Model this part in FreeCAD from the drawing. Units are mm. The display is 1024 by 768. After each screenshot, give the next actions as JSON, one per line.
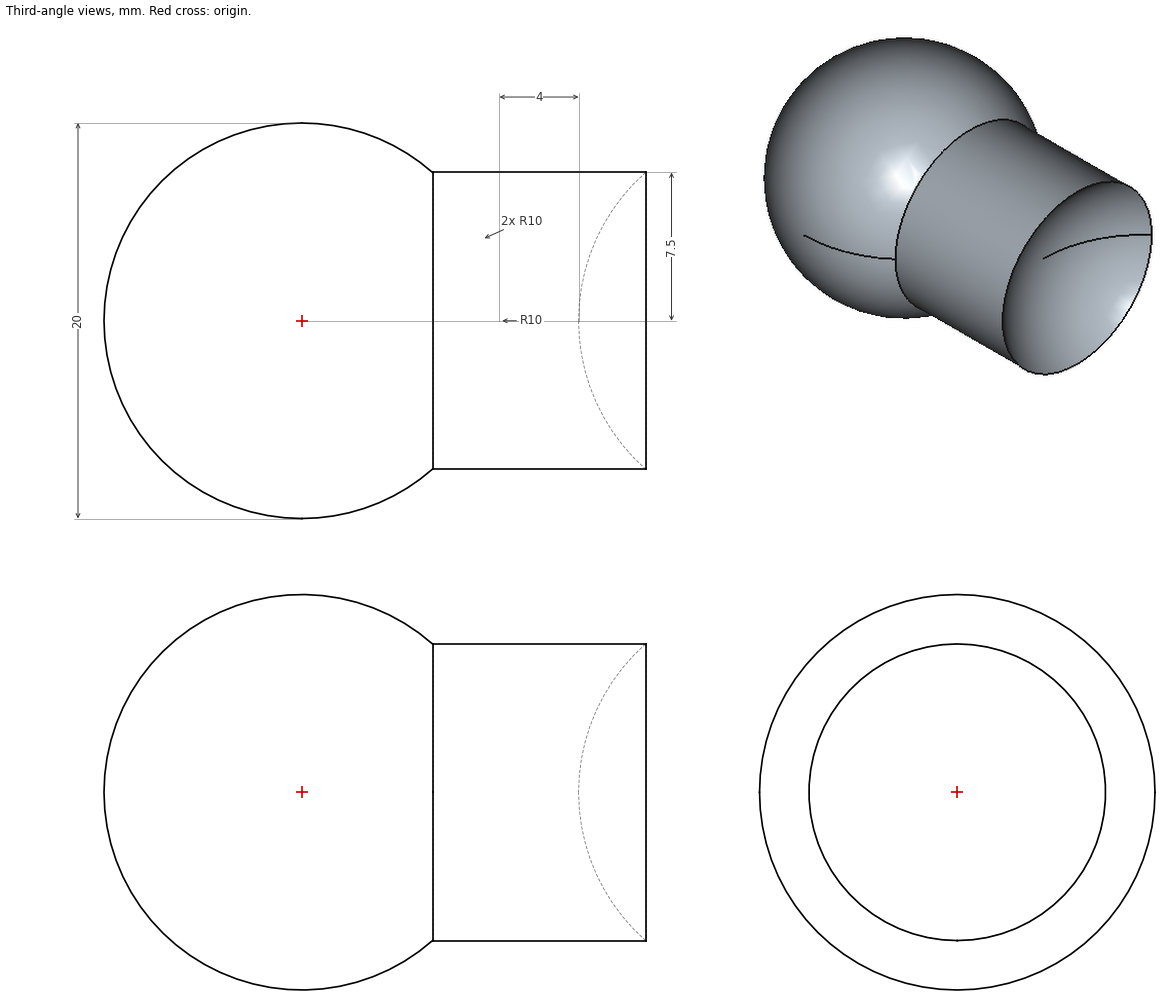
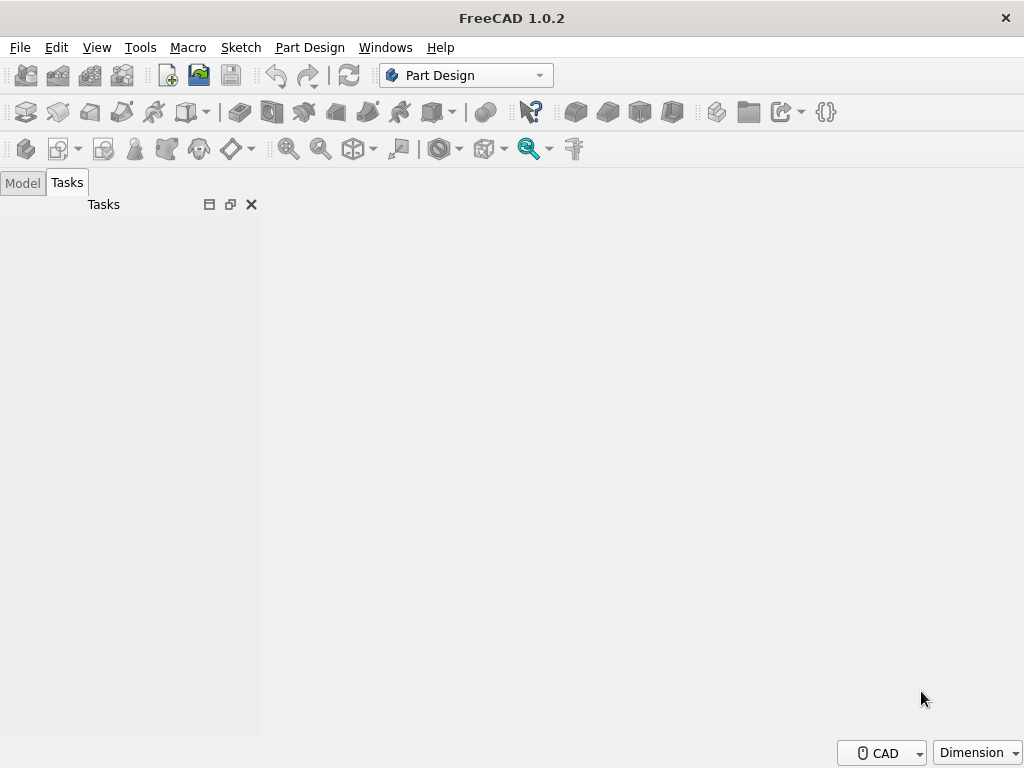
{"action": "key", "text": "ctrl+n"}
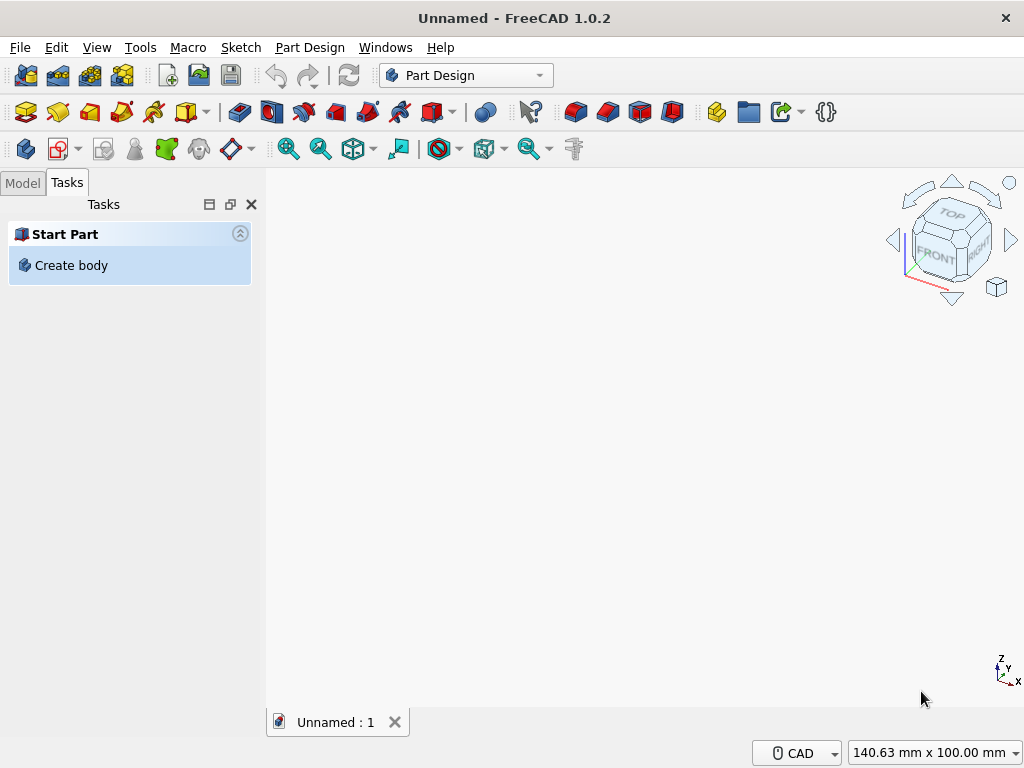
{"action": "left_click", "coordinate": [58, 150]}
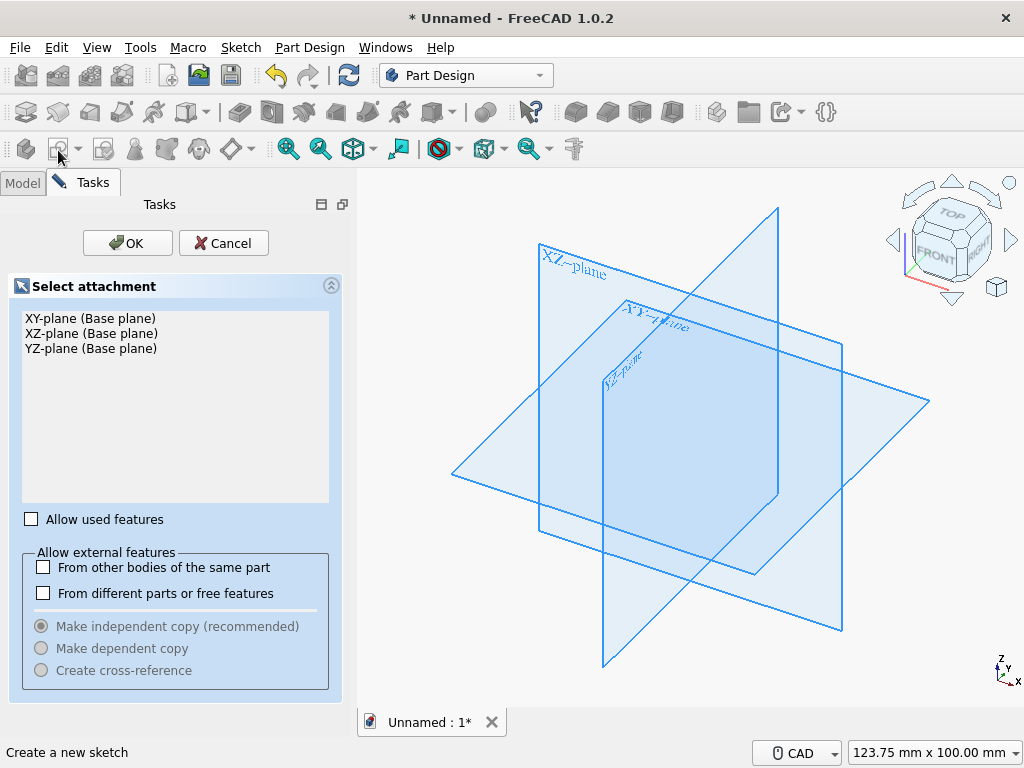
{"action": "left_click", "coordinate": [82, 318]}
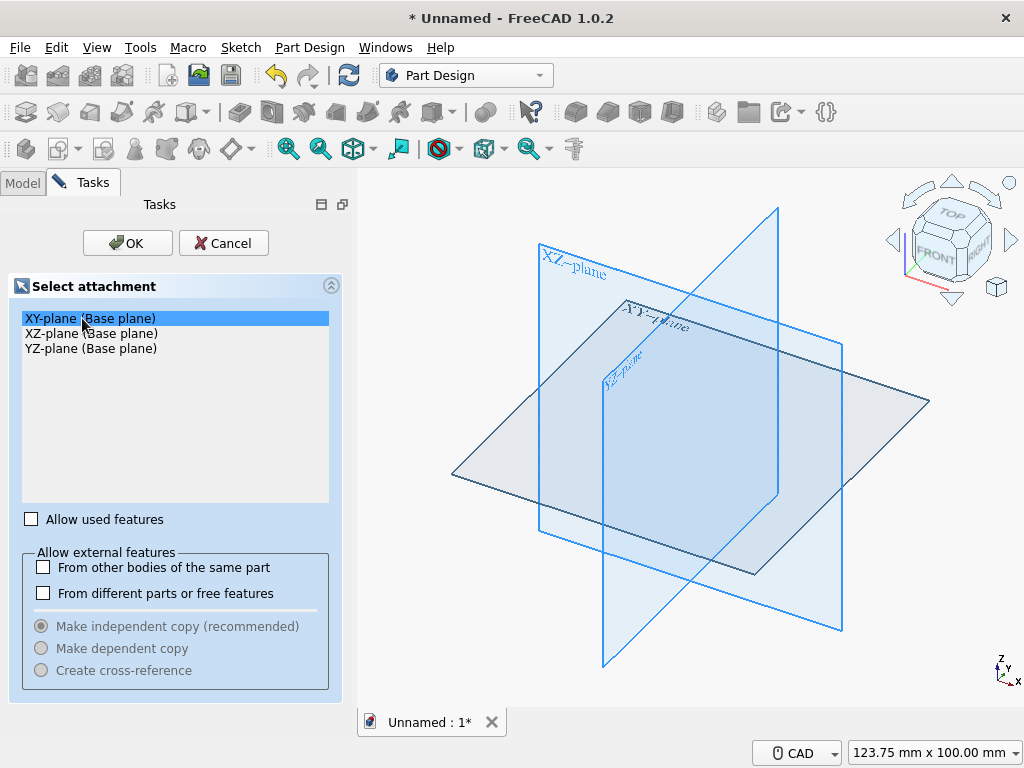
{"action": "left_click", "coordinate": [128, 243]}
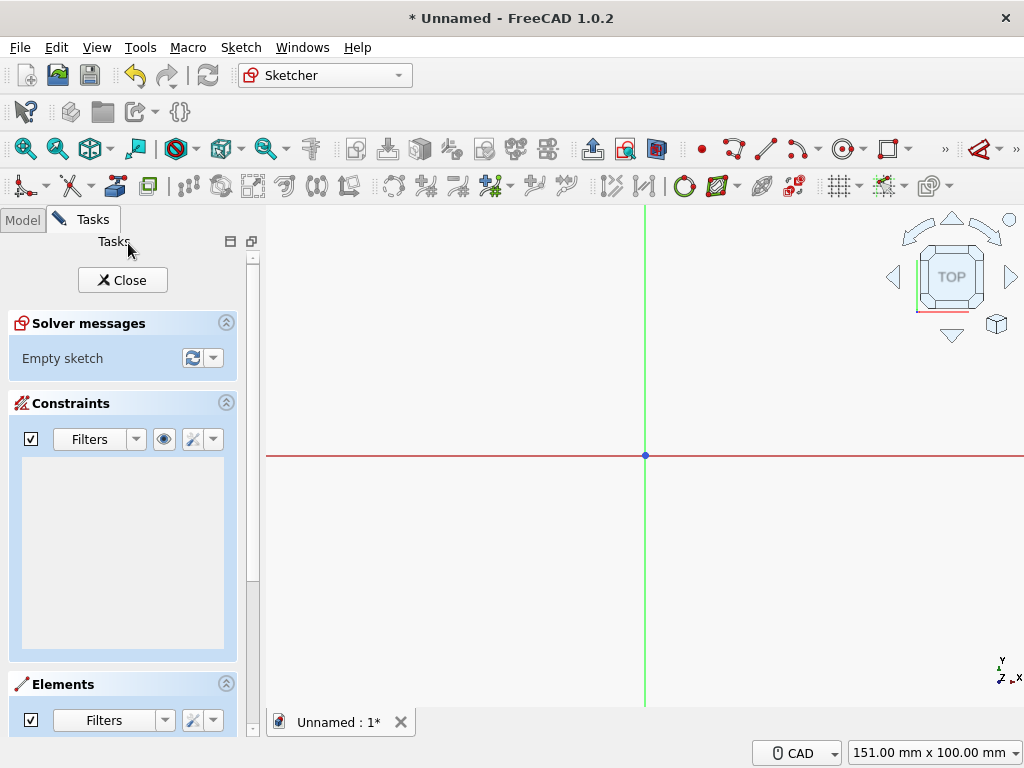
{"action": "scroll", "coordinate": [710, 456], "scroll_direction": "up", "scroll_amount": 6}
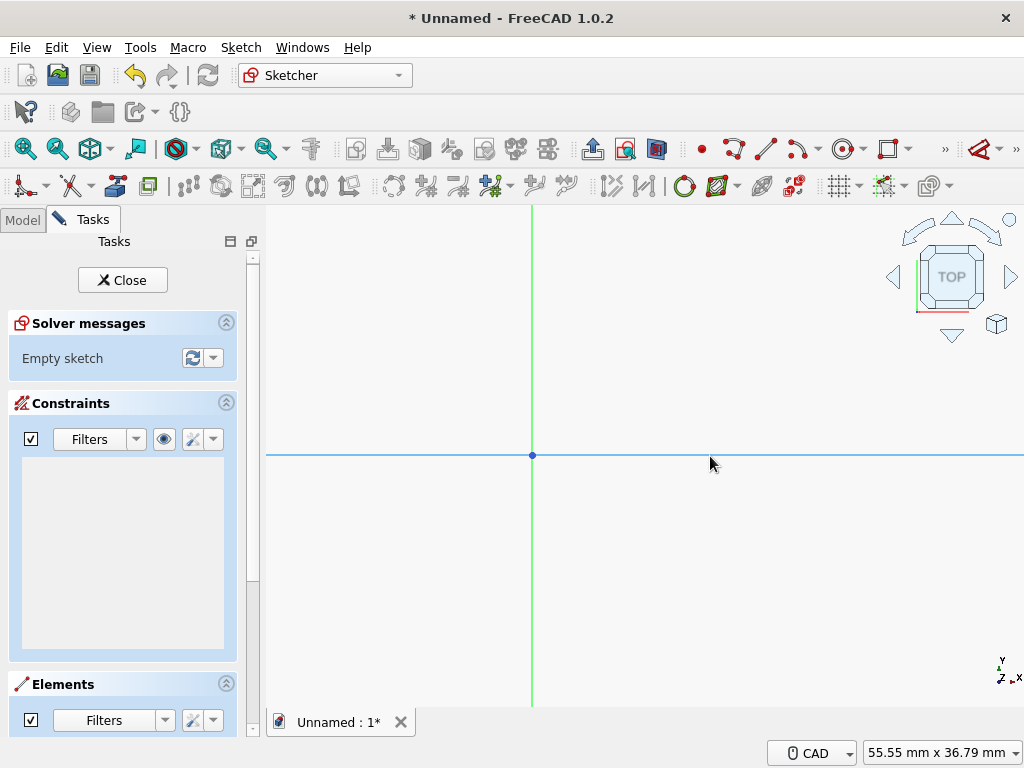
{"action": "key", "text": "g l"}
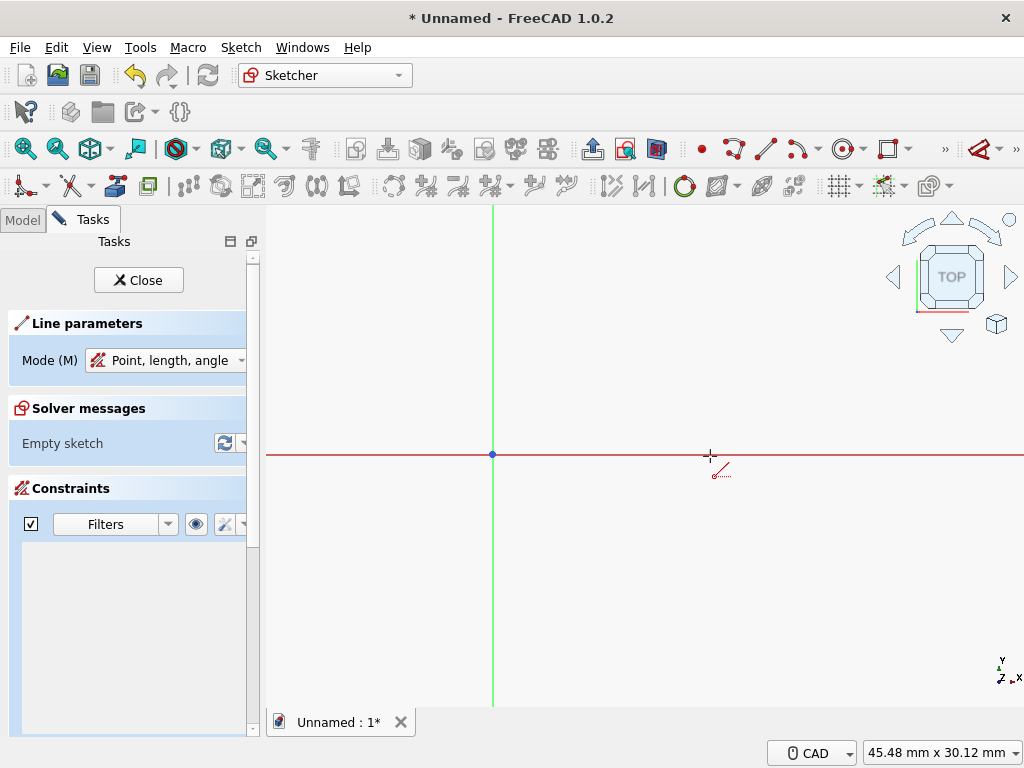
{"action": "left_click", "coordinate": [493, 288]}
{"action": "left_click", "coordinate": [502, 622]}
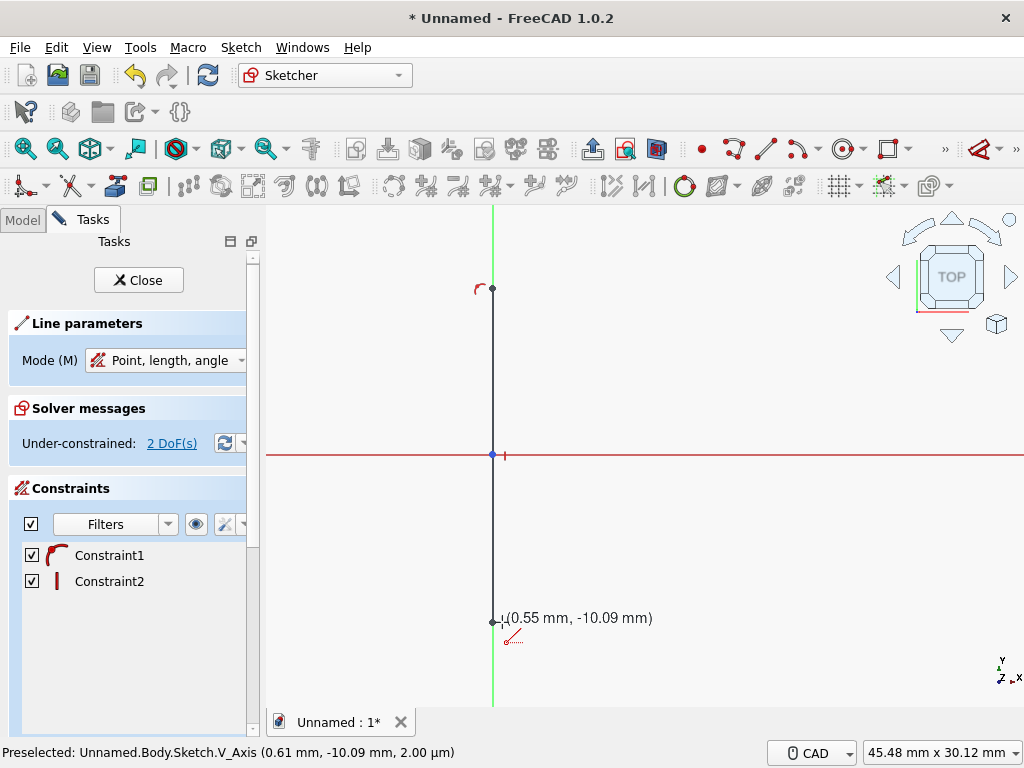
{"action": "key", "text": "g 3 a"}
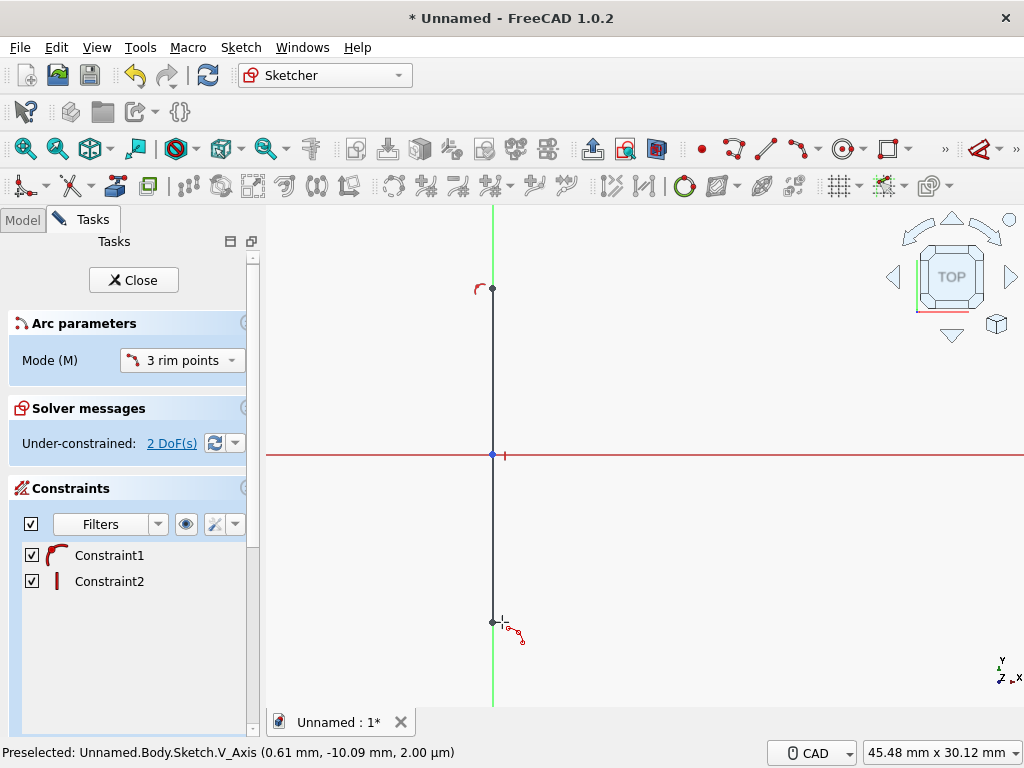
{"action": "left_click", "coordinate": [502, 622]}
{"action": "left_click", "coordinate": [493, 289]}
{"action": "left_click", "coordinate": [651, 506]}
{"action": "key", "text": "Escape"}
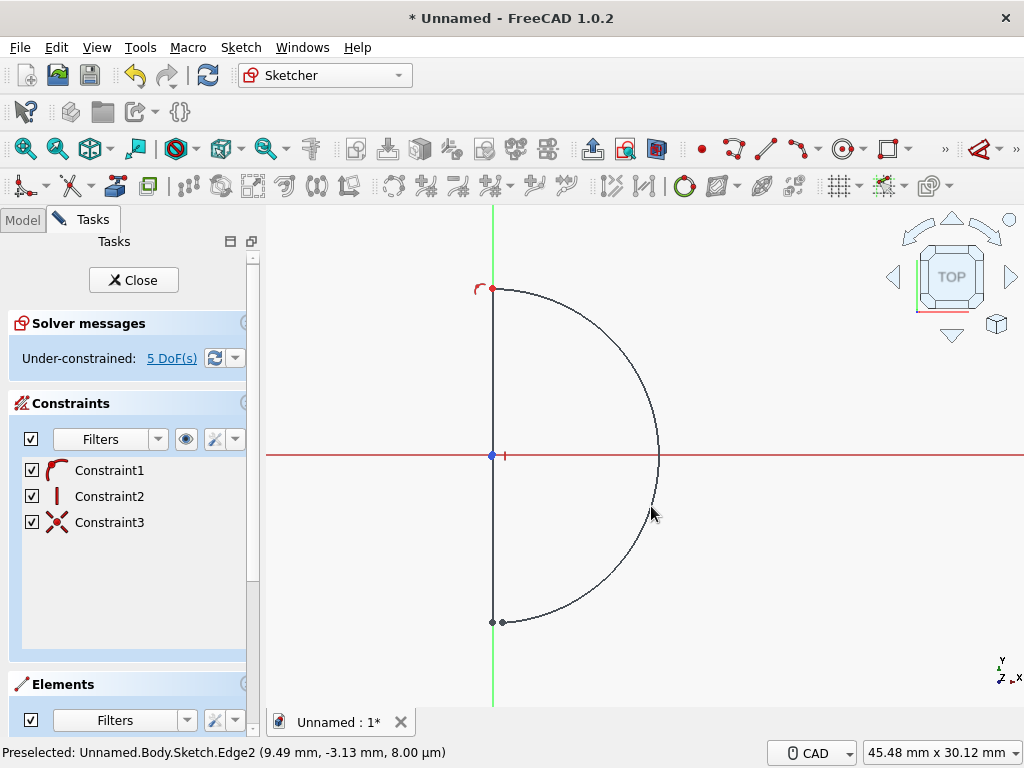
{"action": "left_click_drag", "start_coordinate": [482, 445], "coordinate": [503, 466]}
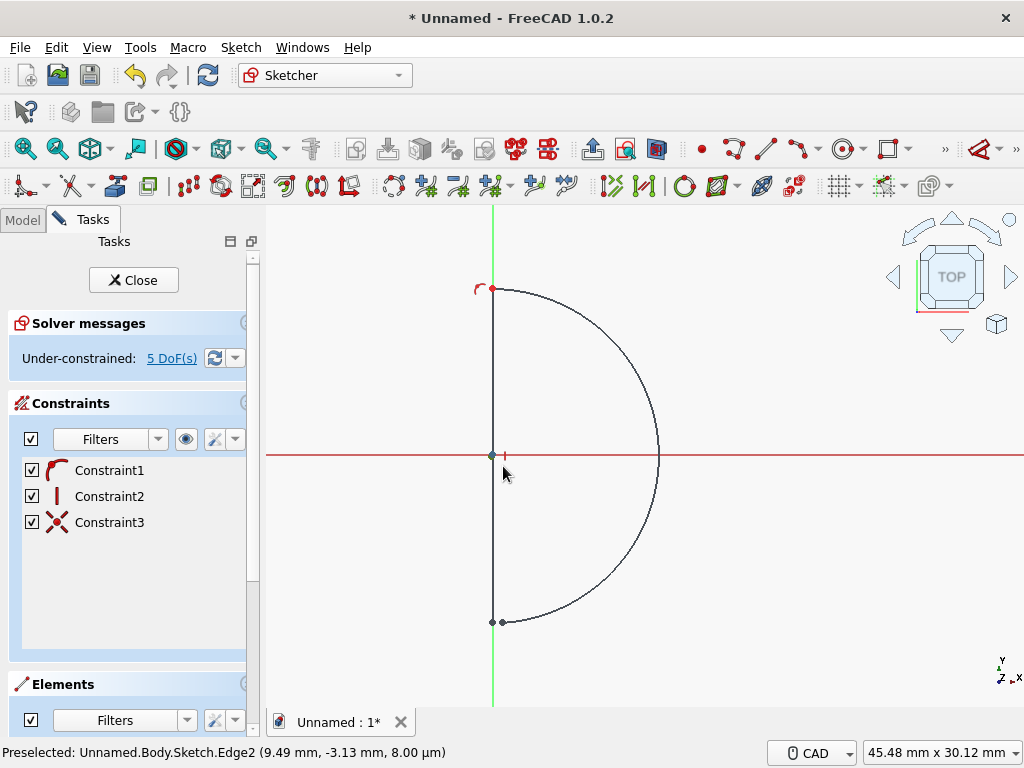
{"action": "key", "text": "c"}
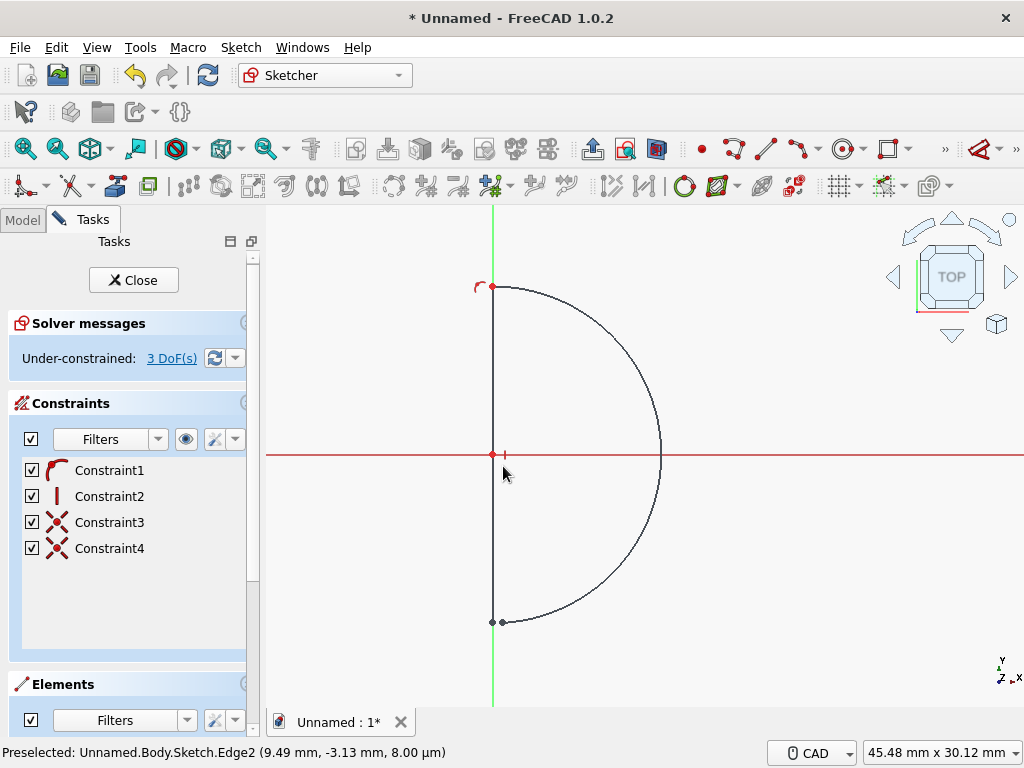
{"action": "left_click", "coordinate": [980, 150]}